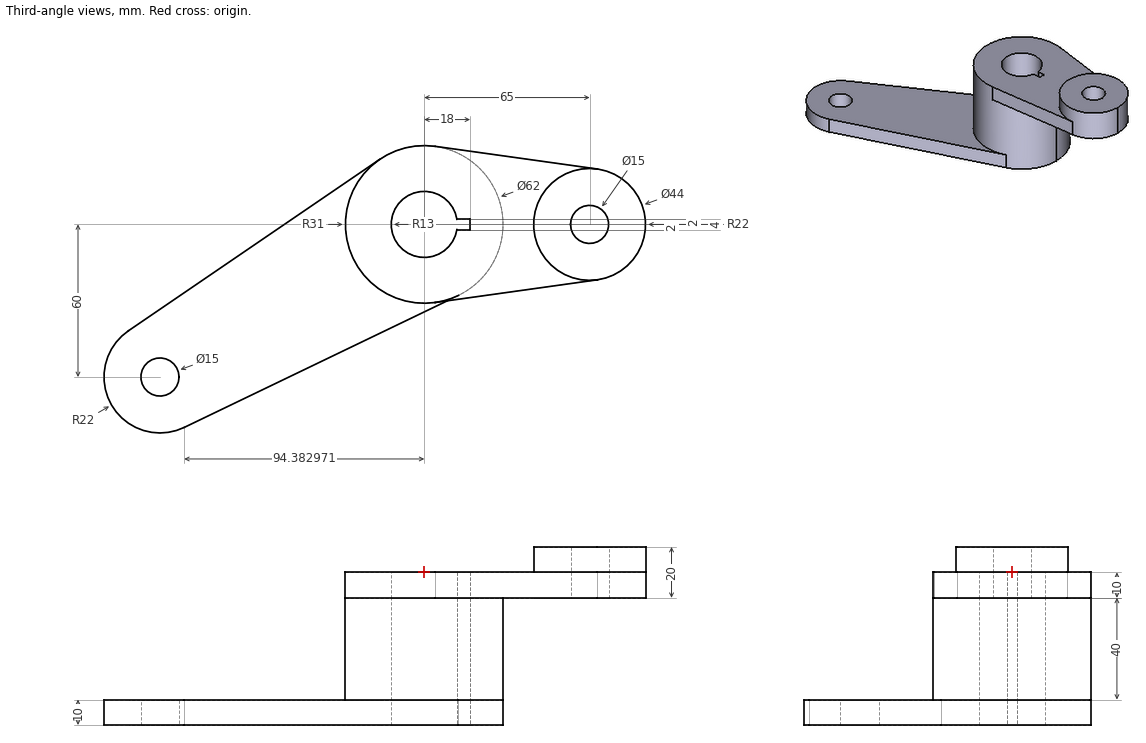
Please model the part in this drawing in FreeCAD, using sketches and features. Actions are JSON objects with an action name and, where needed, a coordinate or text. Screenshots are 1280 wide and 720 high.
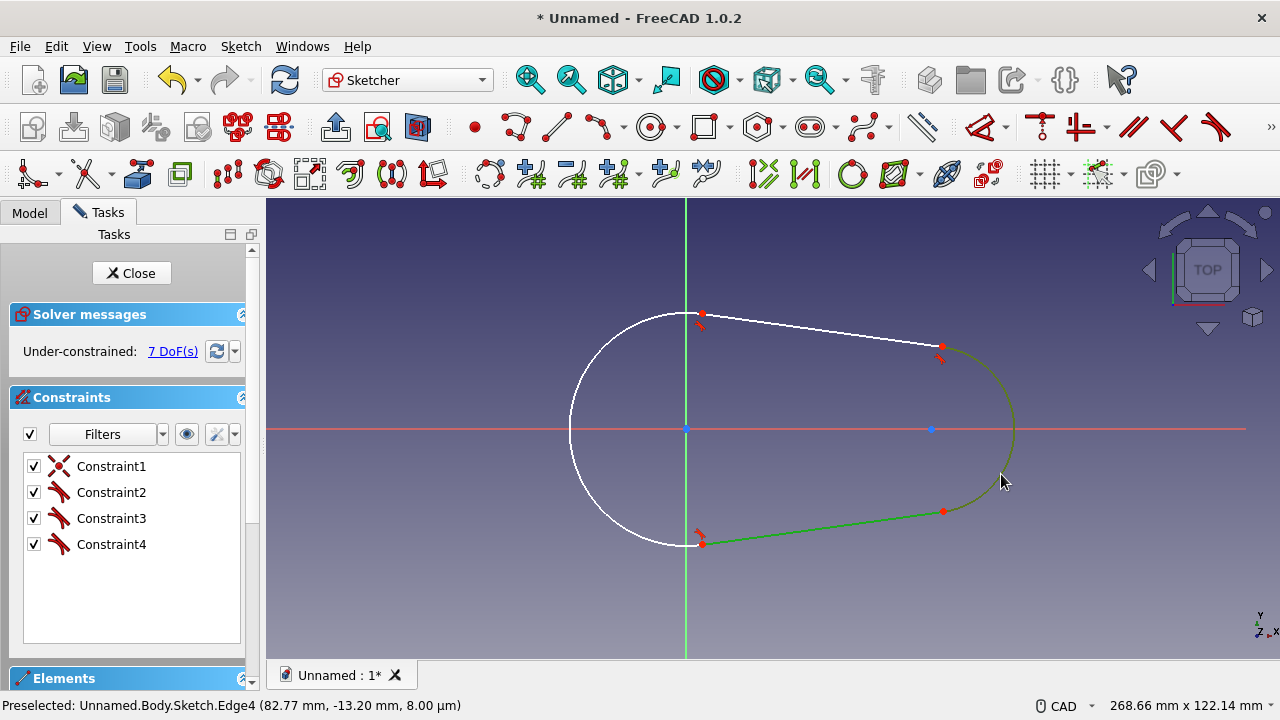
{"action": "key", "text": "t"}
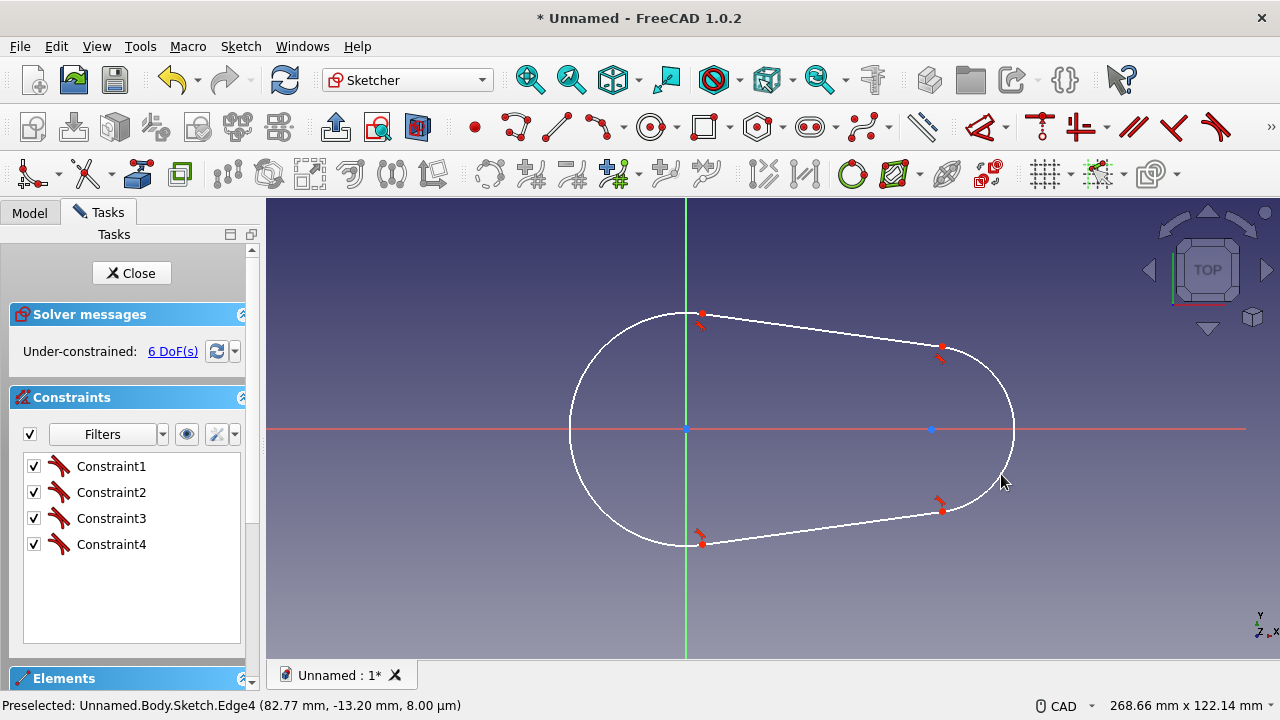
{"action": "left_click_drag", "start_coordinate": [676, 418], "coordinate": [696, 440]}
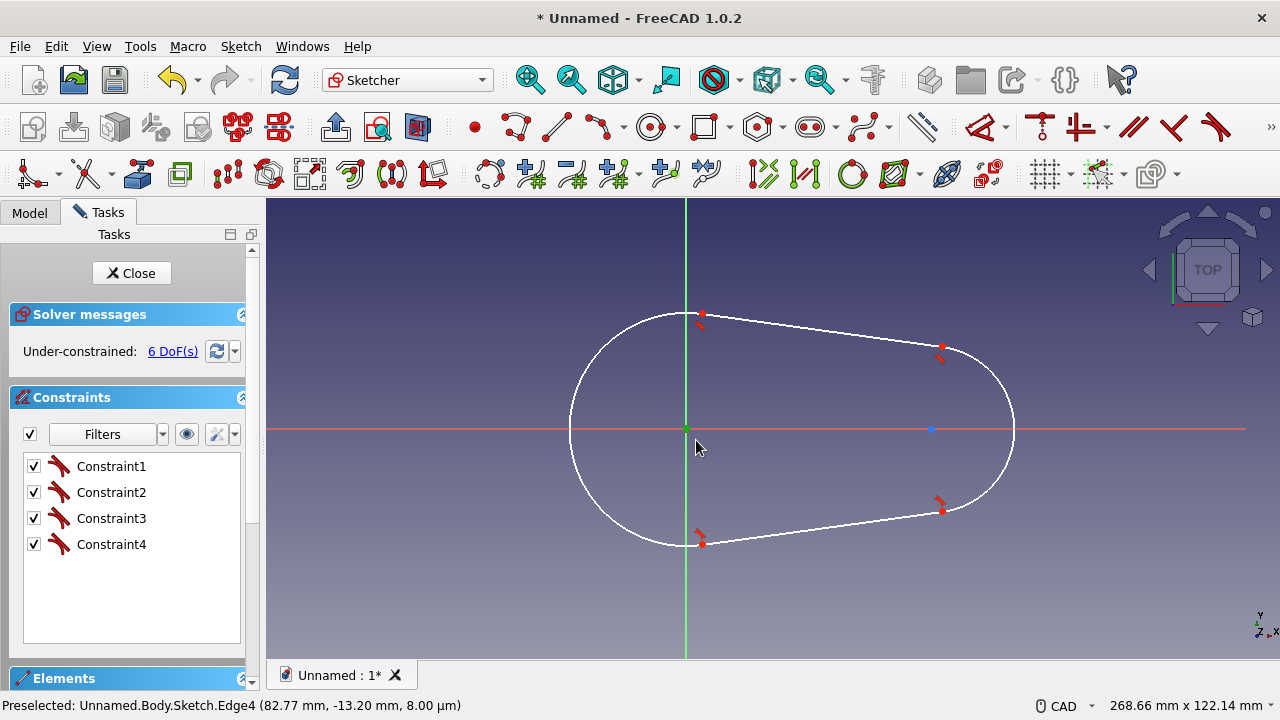
{"action": "left_click", "coordinate": [1040, 128]}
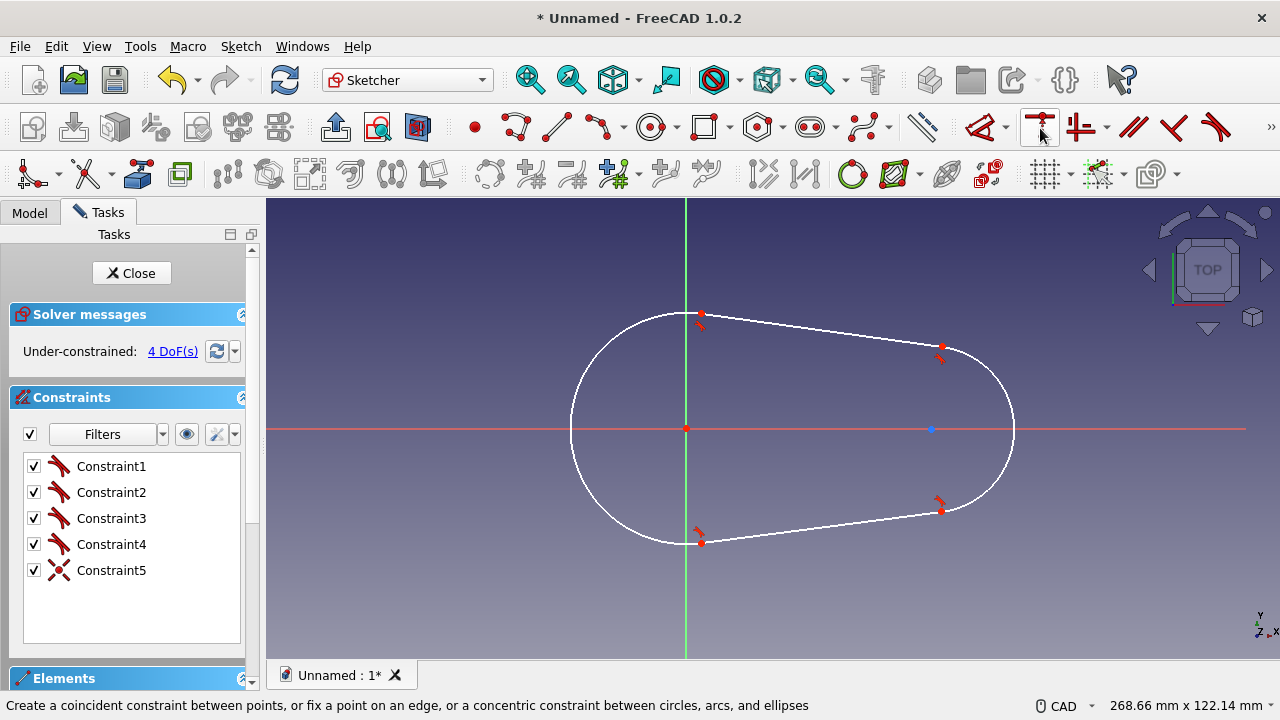
{"action": "left_click", "coordinate": [931, 429]}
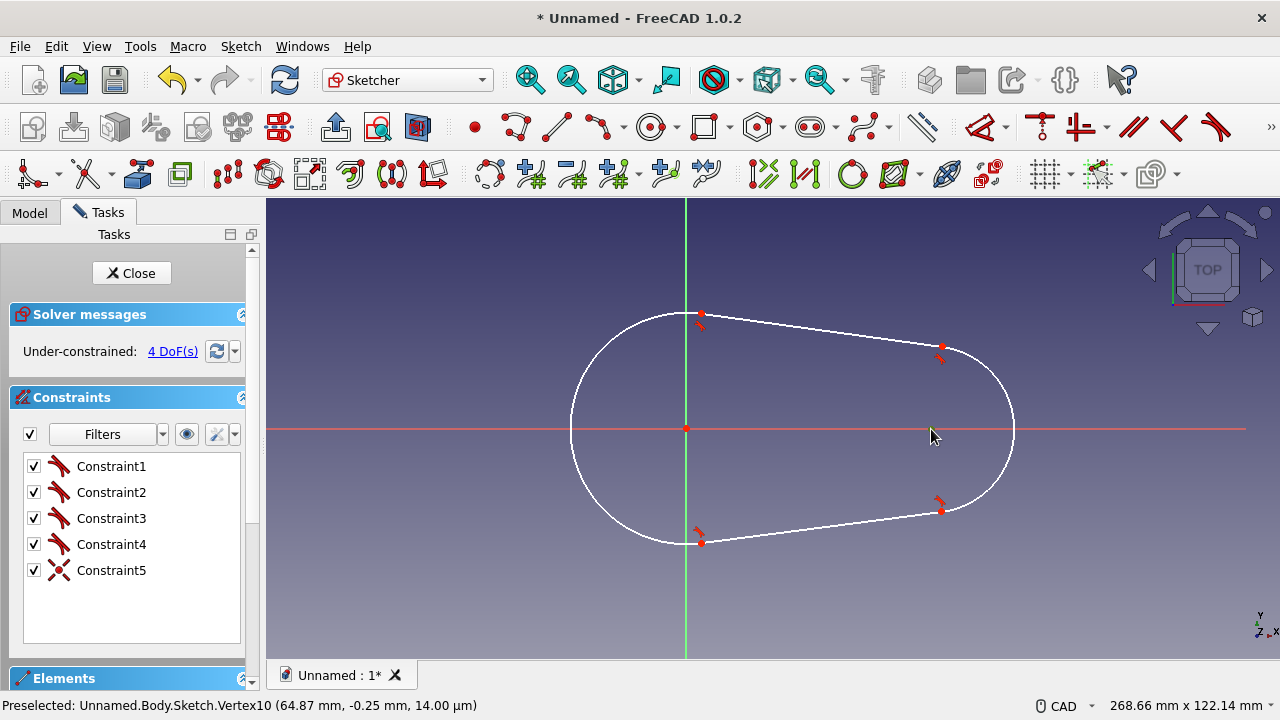
{"action": "left_click", "coordinate": [353, 428]}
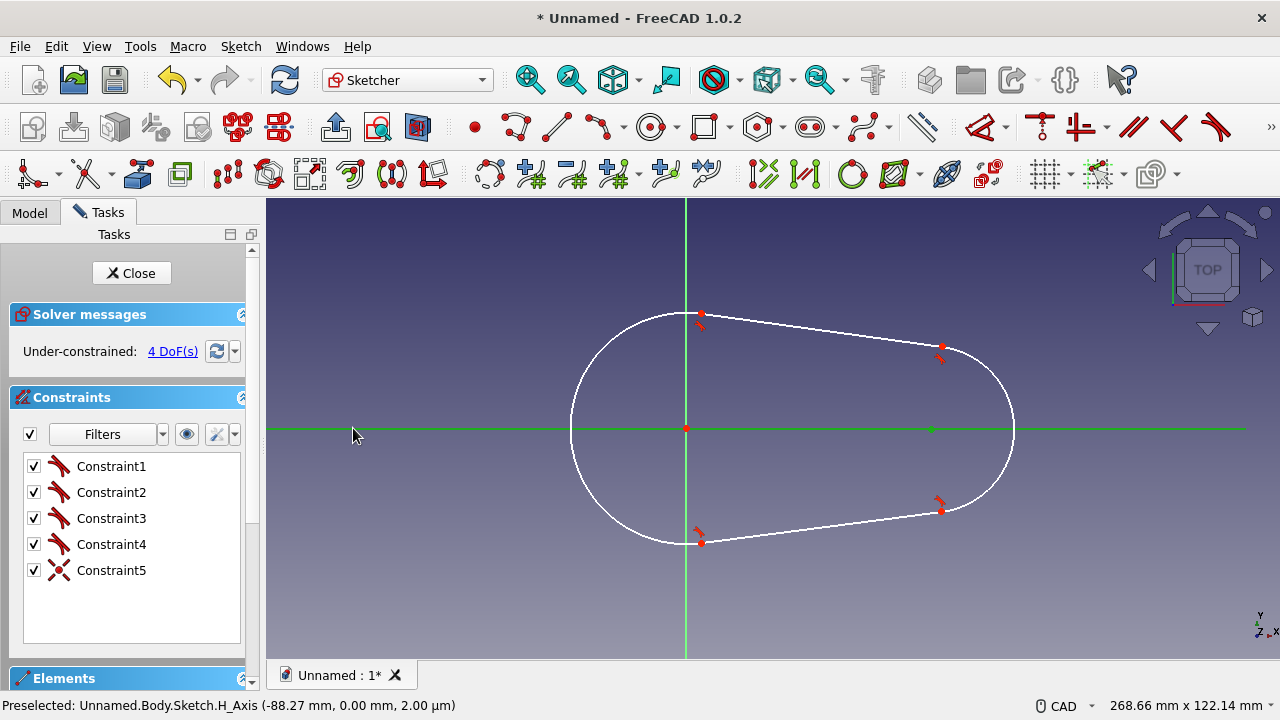
{"action": "key", "text": "c"}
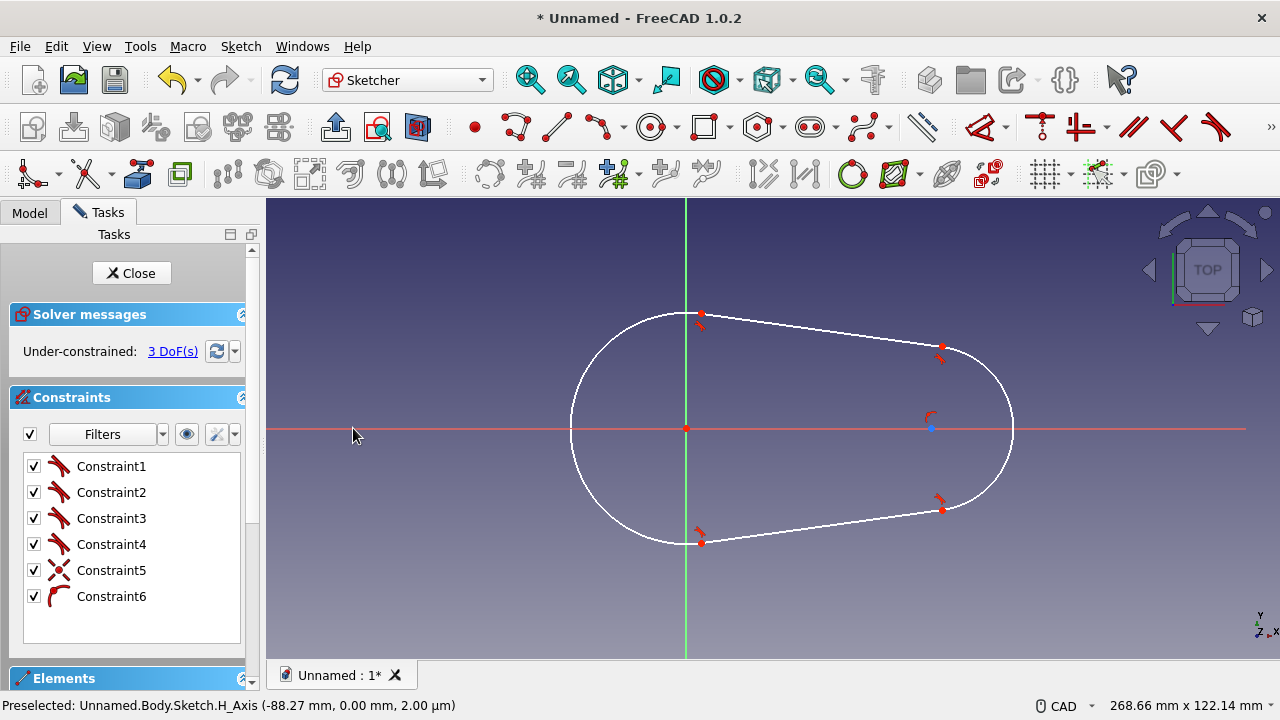
{"action": "key", "text": "d"}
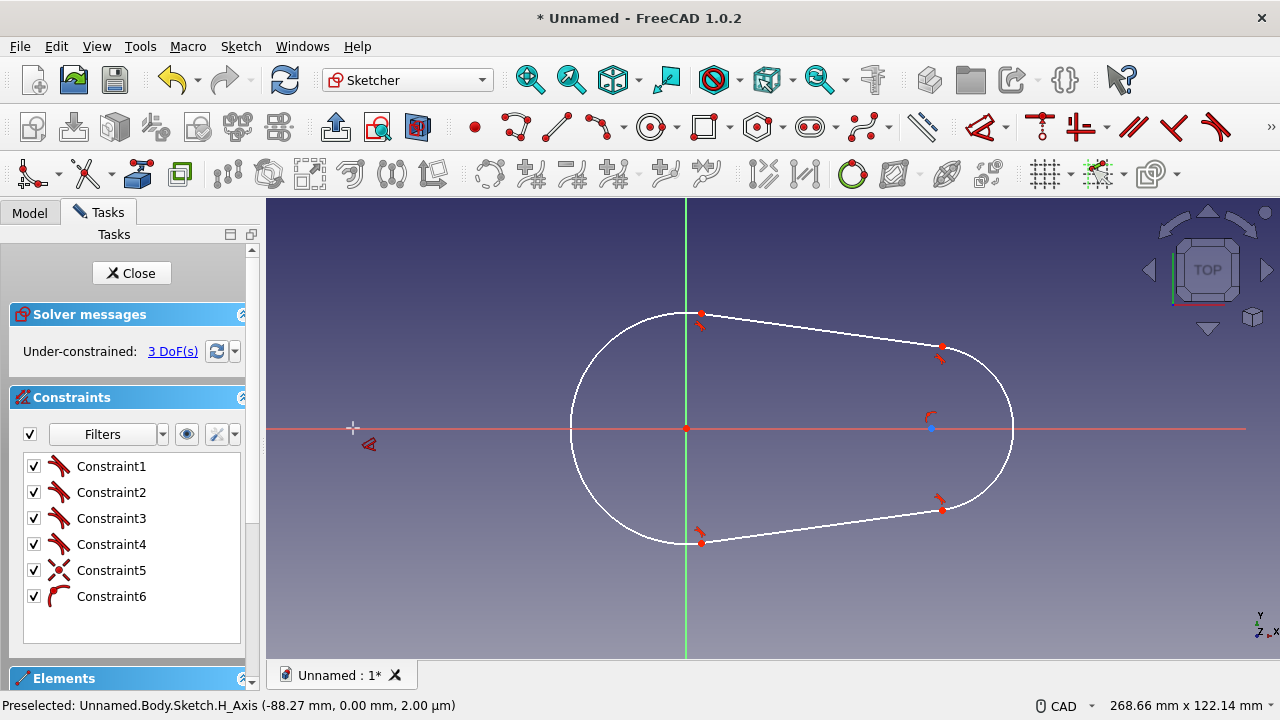
{"action": "left_click", "coordinate": [596, 355]}
{"action": "left_click", "coordinate": [571, 335]}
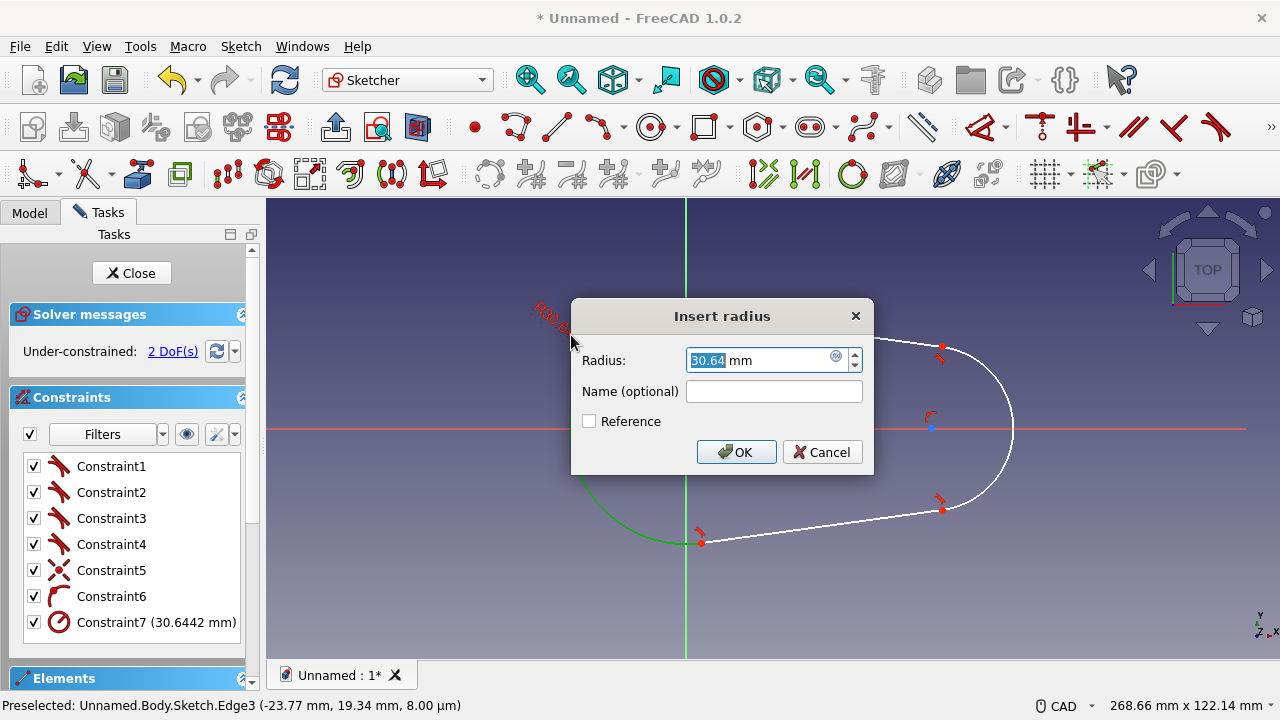
{"action": "type", "text": "31"}
{"action": "key", "text": "Return"}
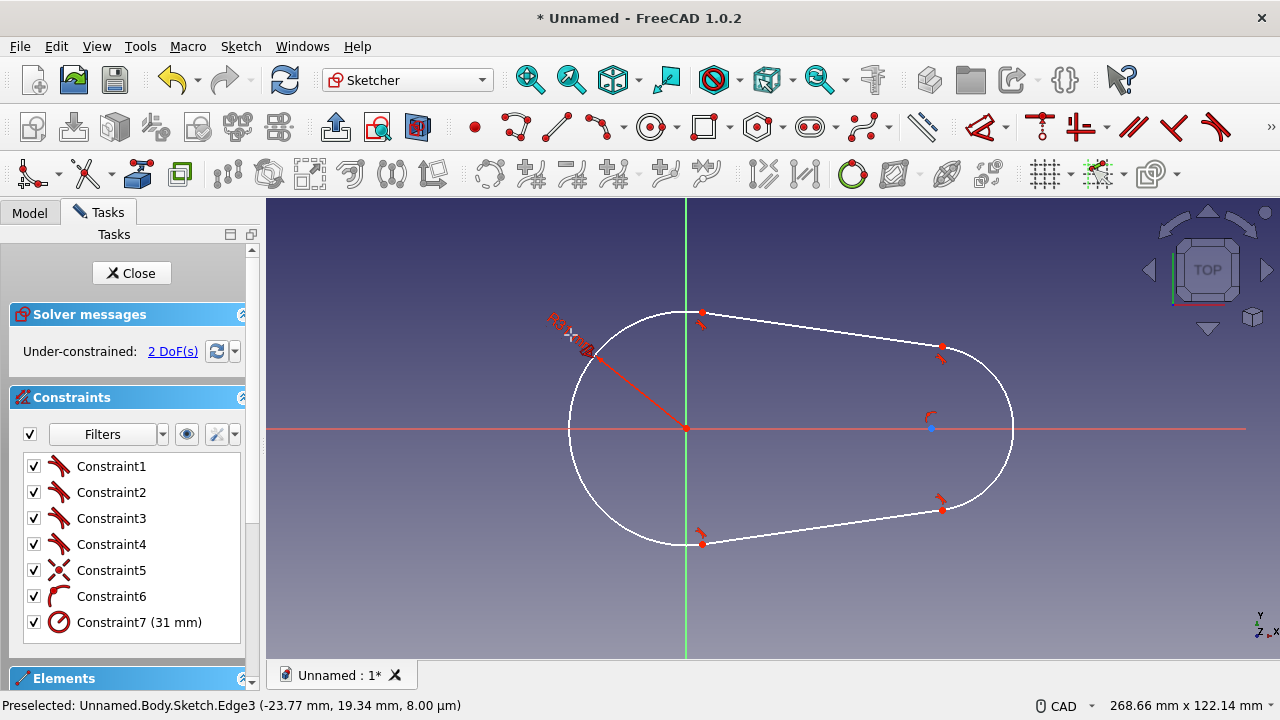
{"action": "left_click", "coordinate": [1000, 473]}
{"action": "left_click", "coordinate": [1027, 490]}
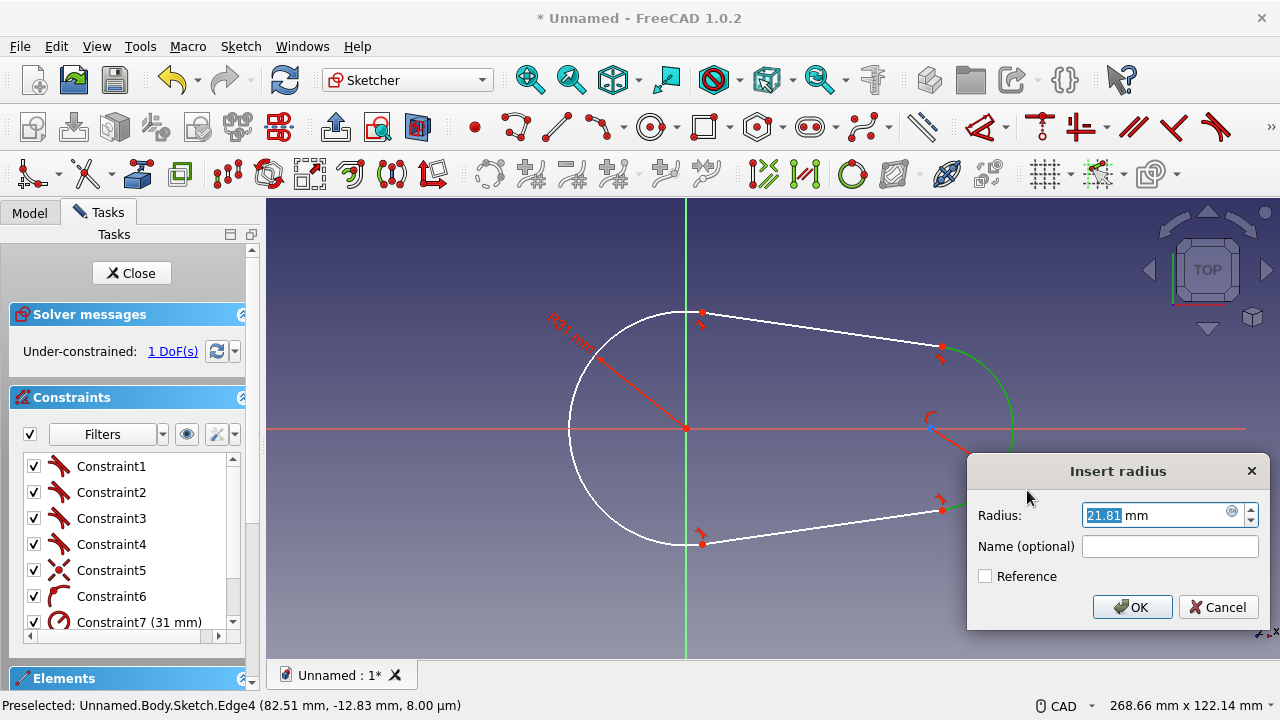
{"action": "type", "text": "22"}
{"action": "key", "text": "Return"}